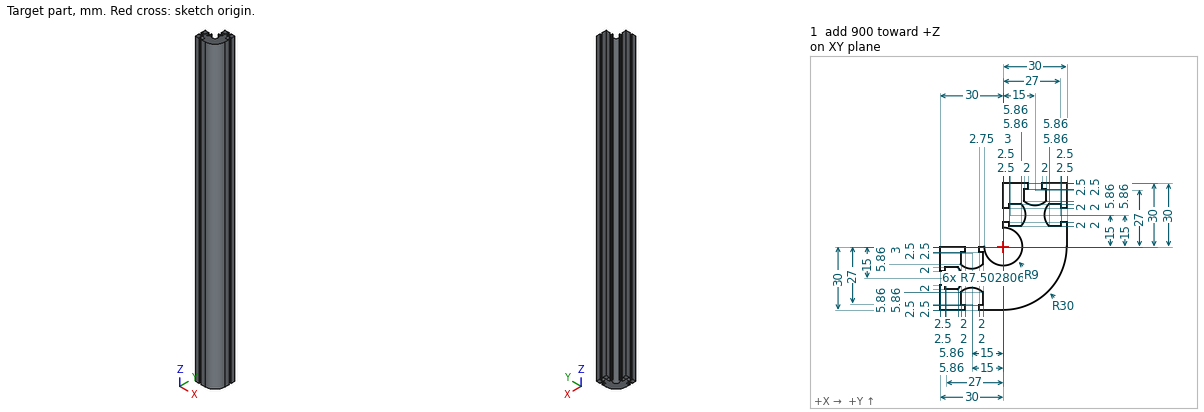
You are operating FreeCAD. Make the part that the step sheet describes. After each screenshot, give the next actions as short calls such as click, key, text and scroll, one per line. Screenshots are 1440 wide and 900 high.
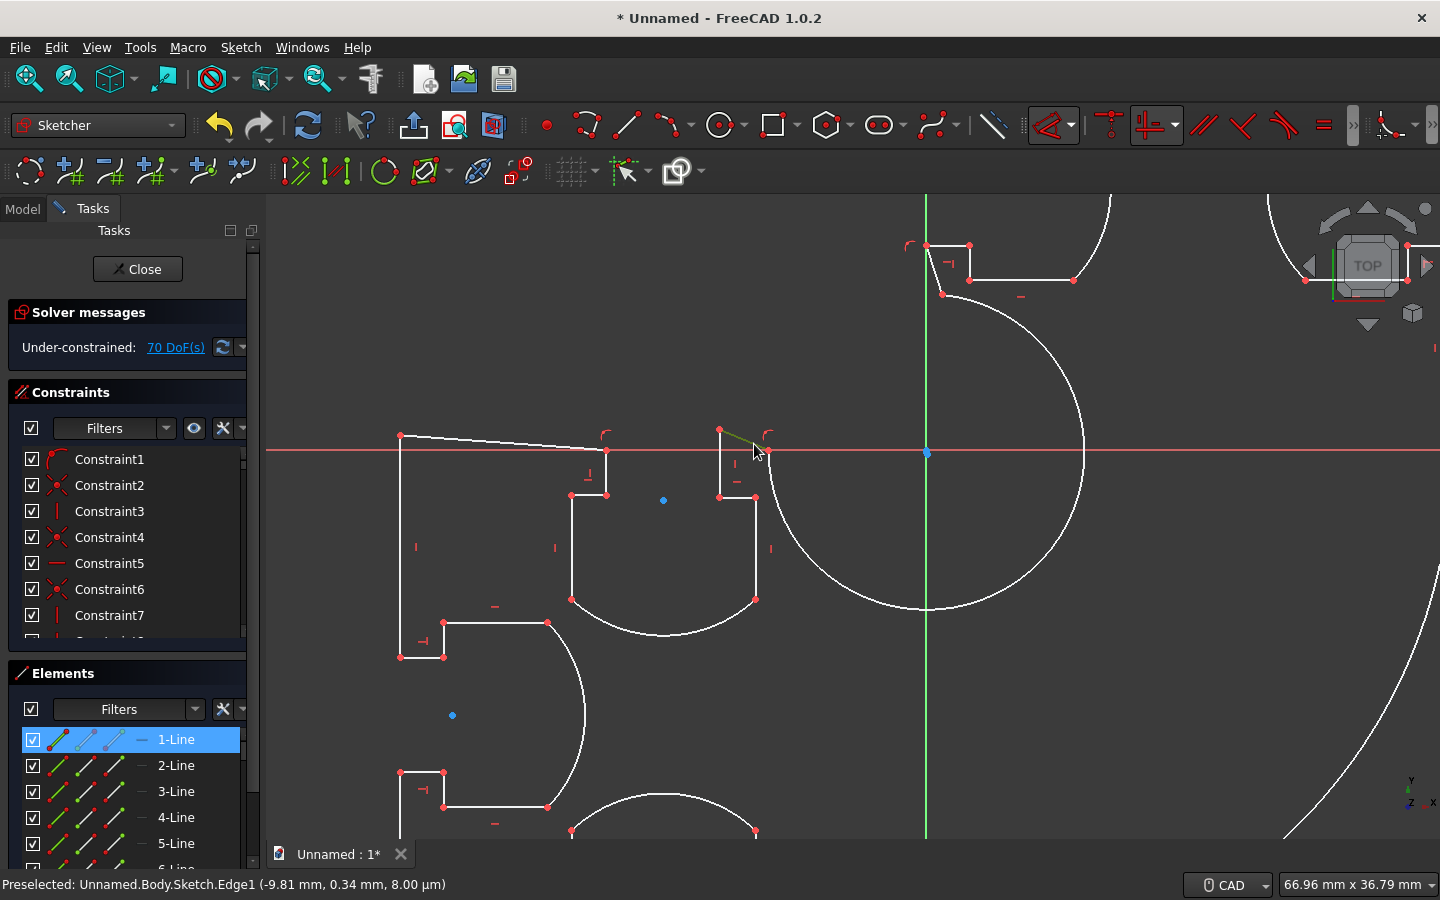
key(h)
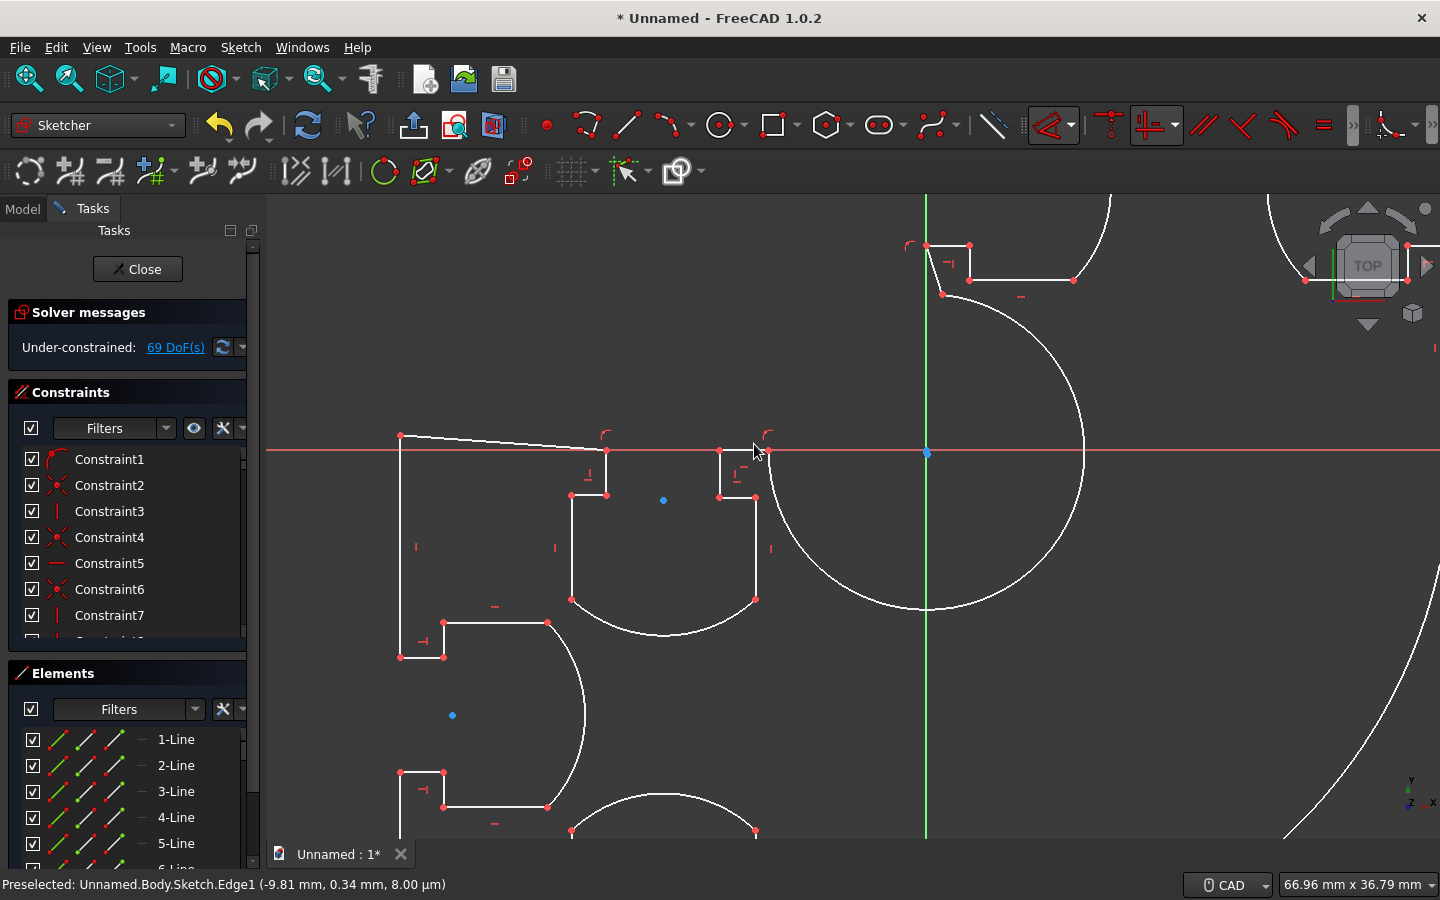
scroll(462, 440, up, 2)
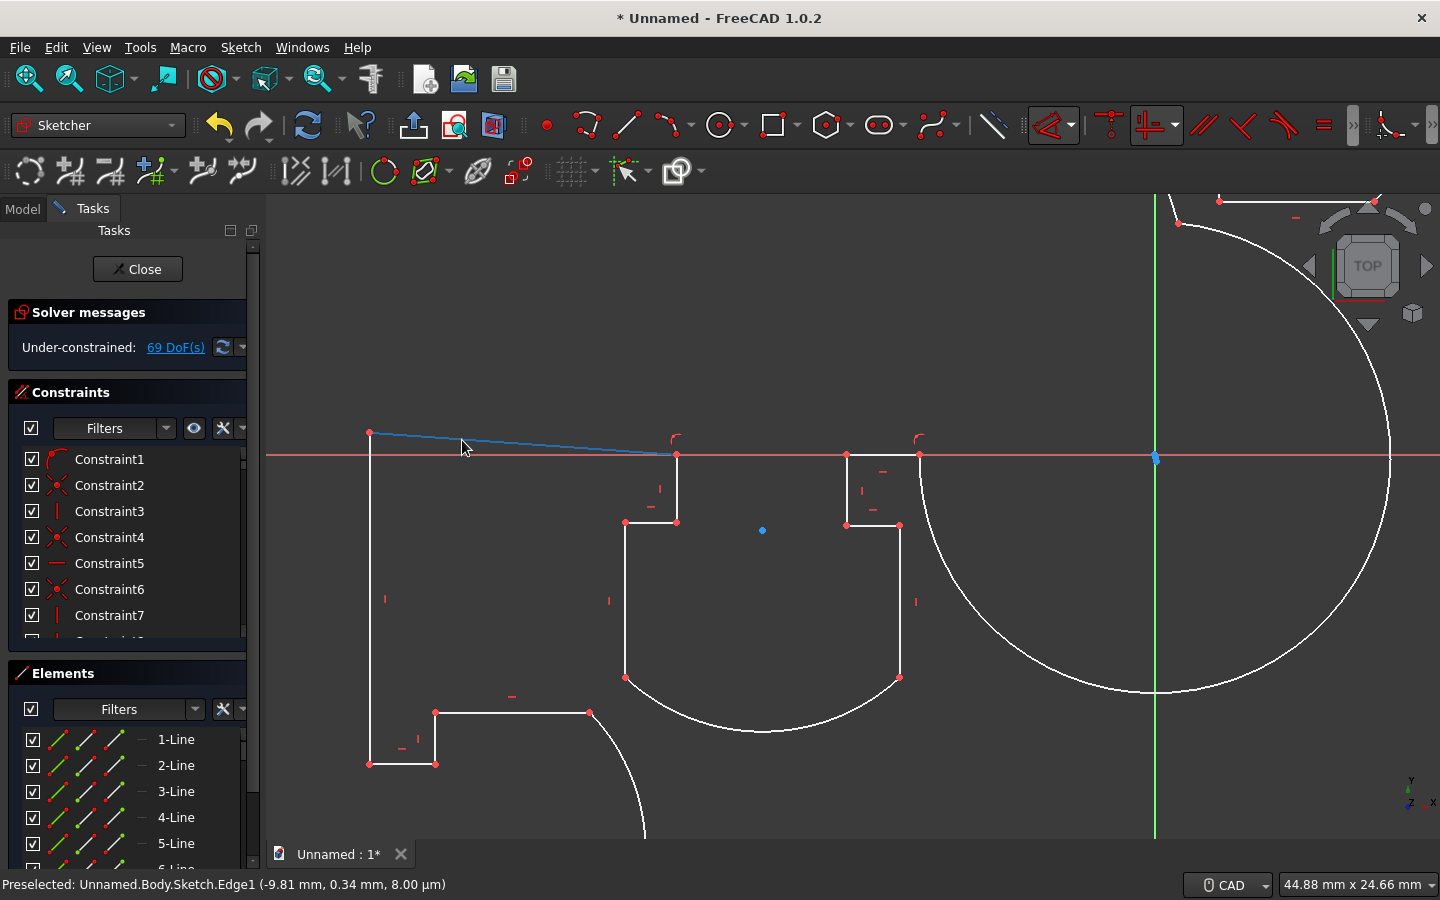
click(462, 439)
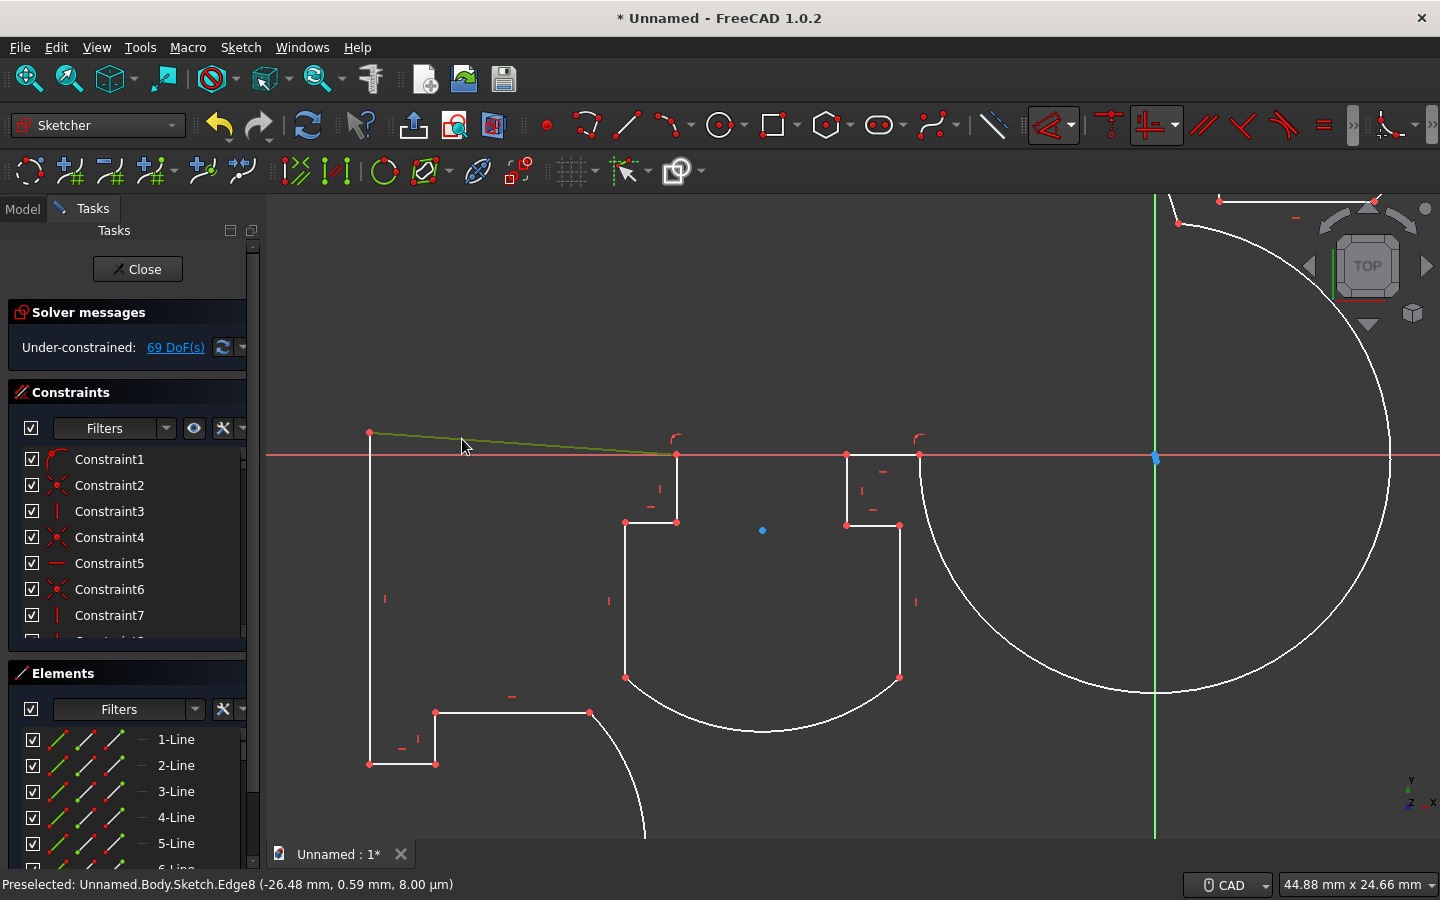
key(h)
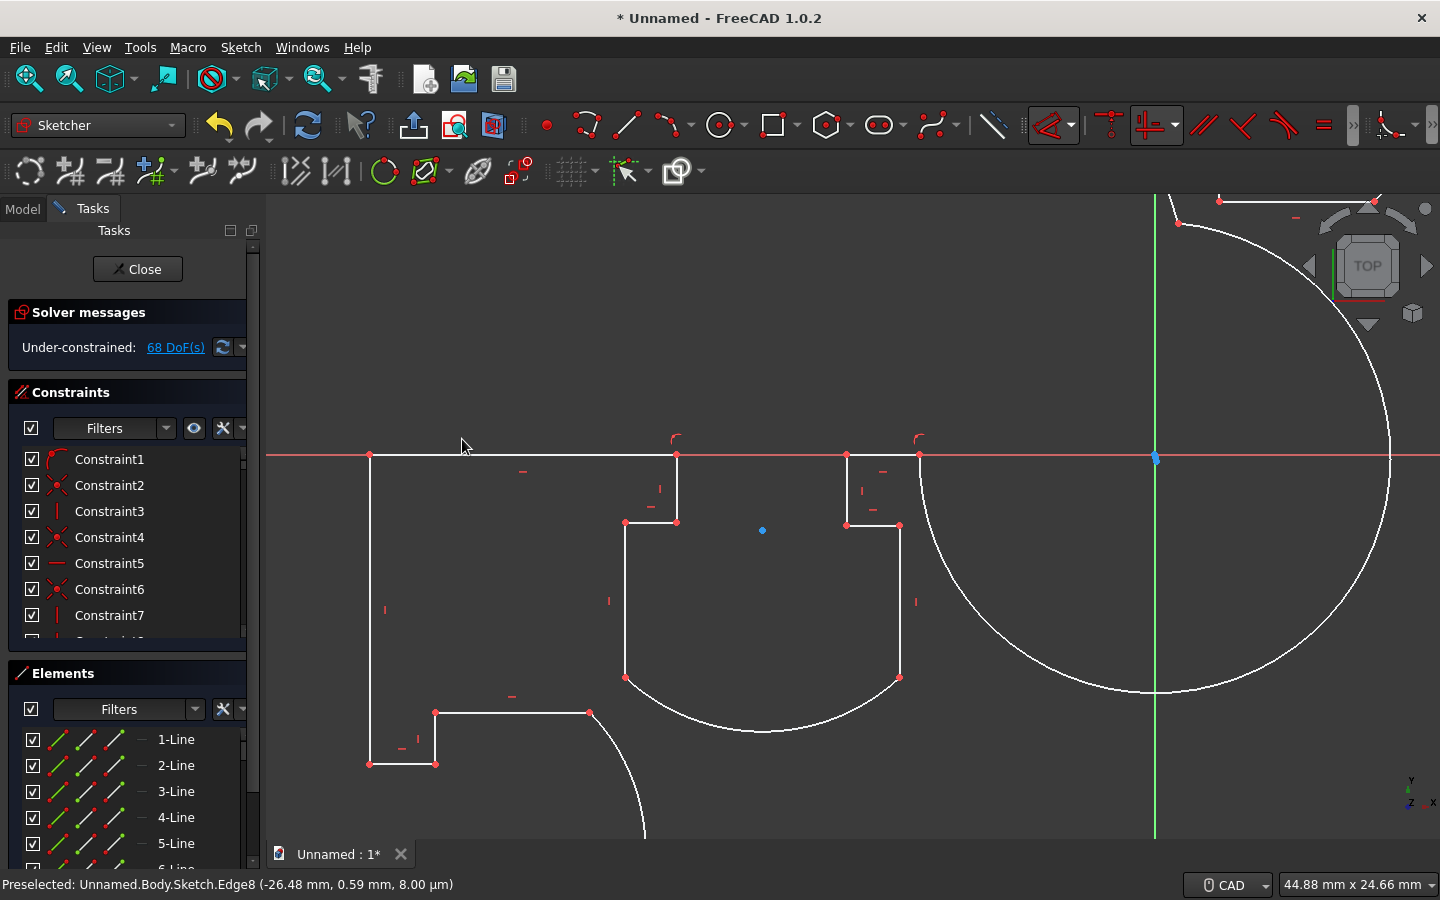
scroll(663, 537, down, 7)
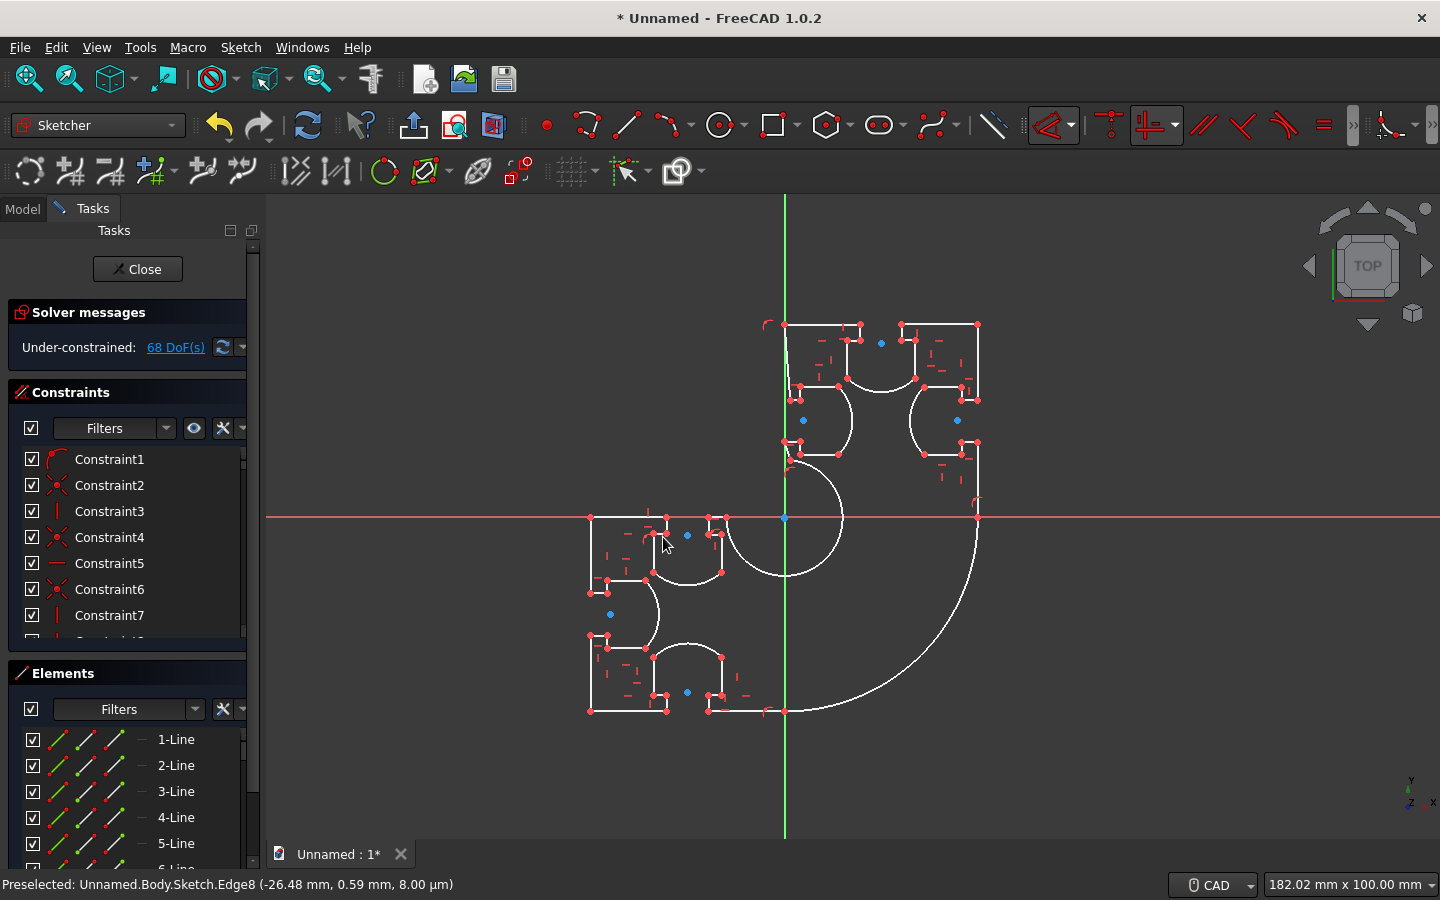
scroll(789, 378, up, 7)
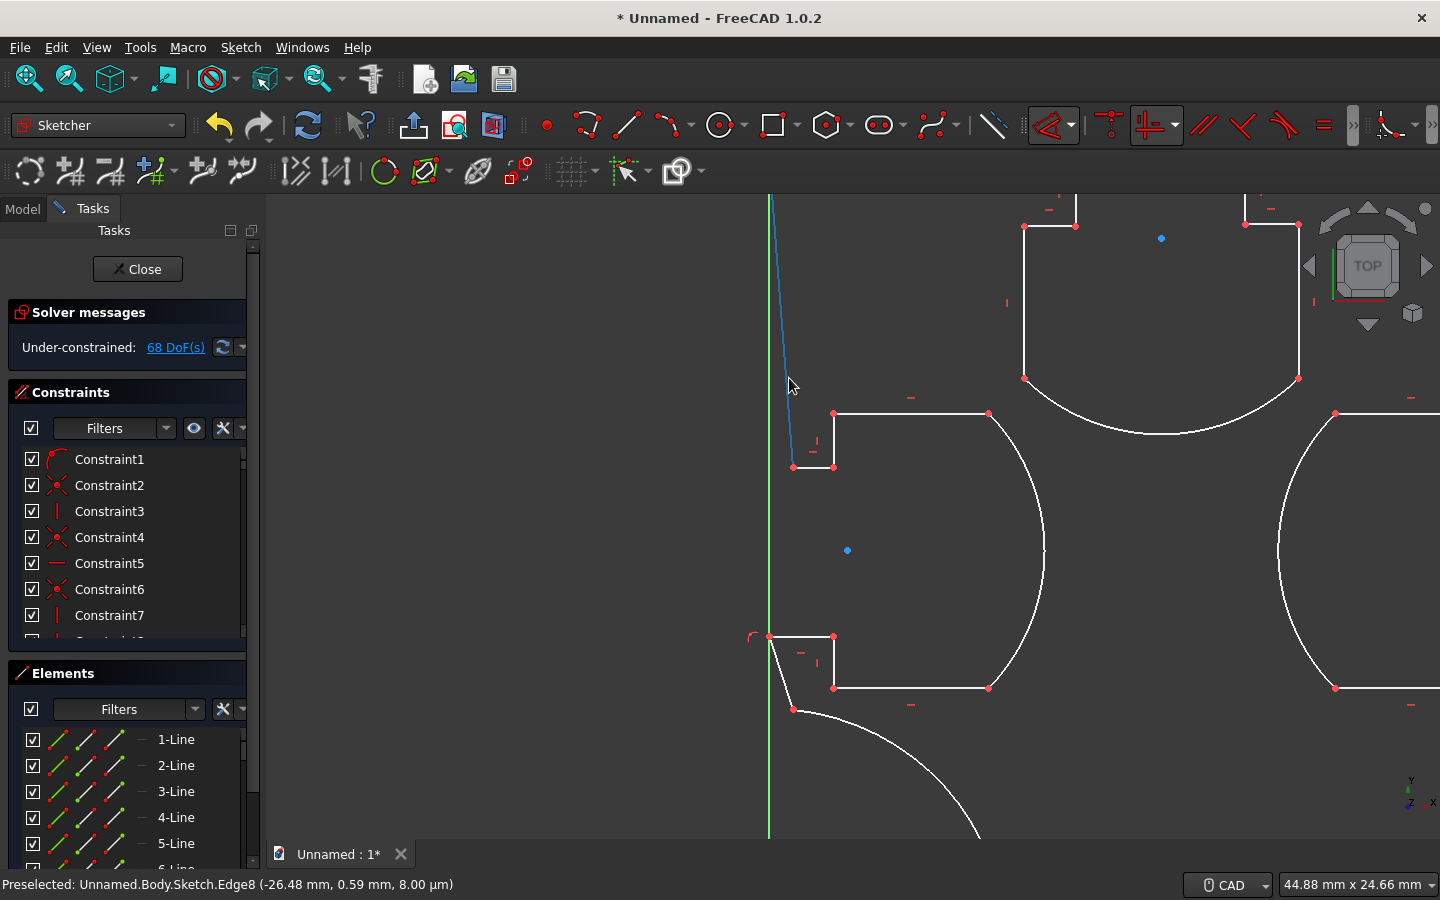
click(786, 376)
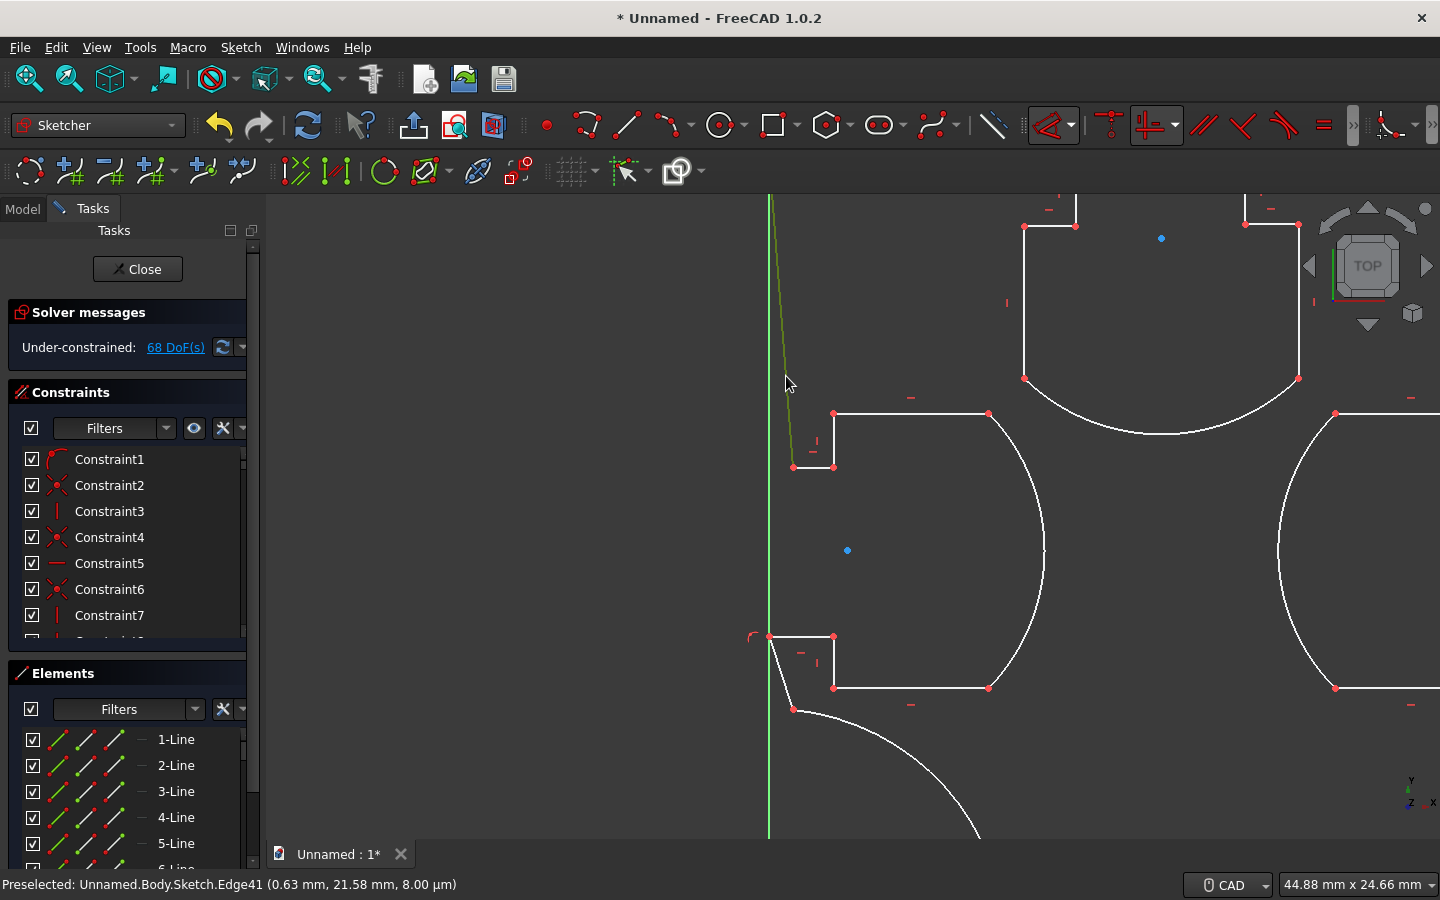
click(1178, 126)